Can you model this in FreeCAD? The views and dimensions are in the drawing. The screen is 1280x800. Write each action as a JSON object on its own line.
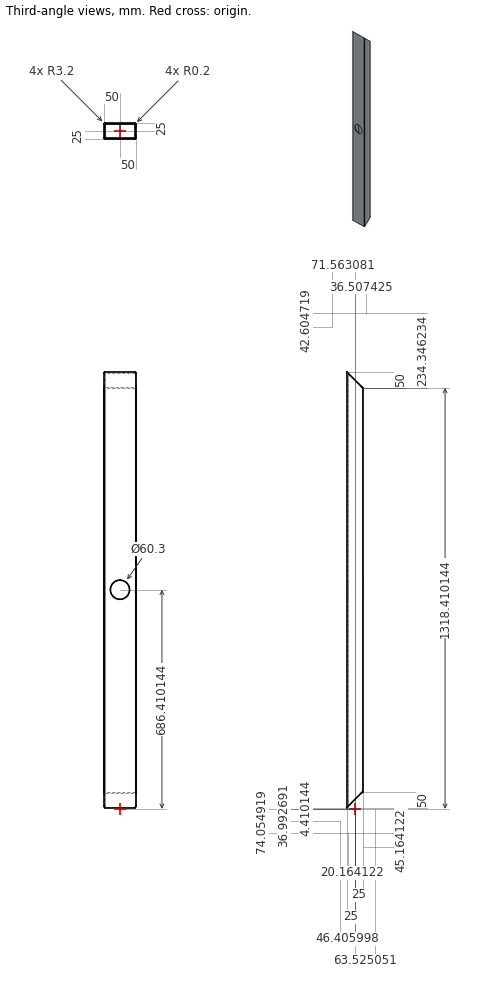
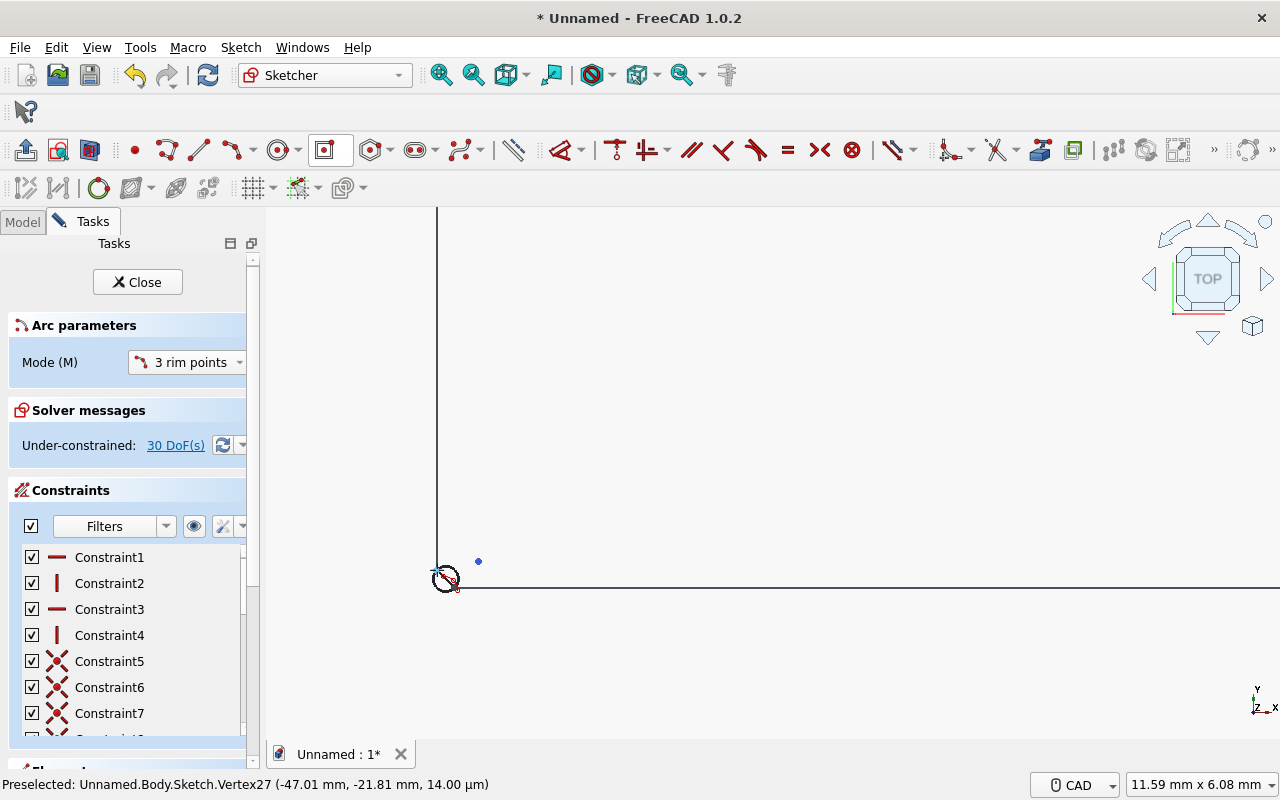
{"action": "scroll", "coordinate": [442, 582], "scroll_direction": "up", "scroll_amount": 6}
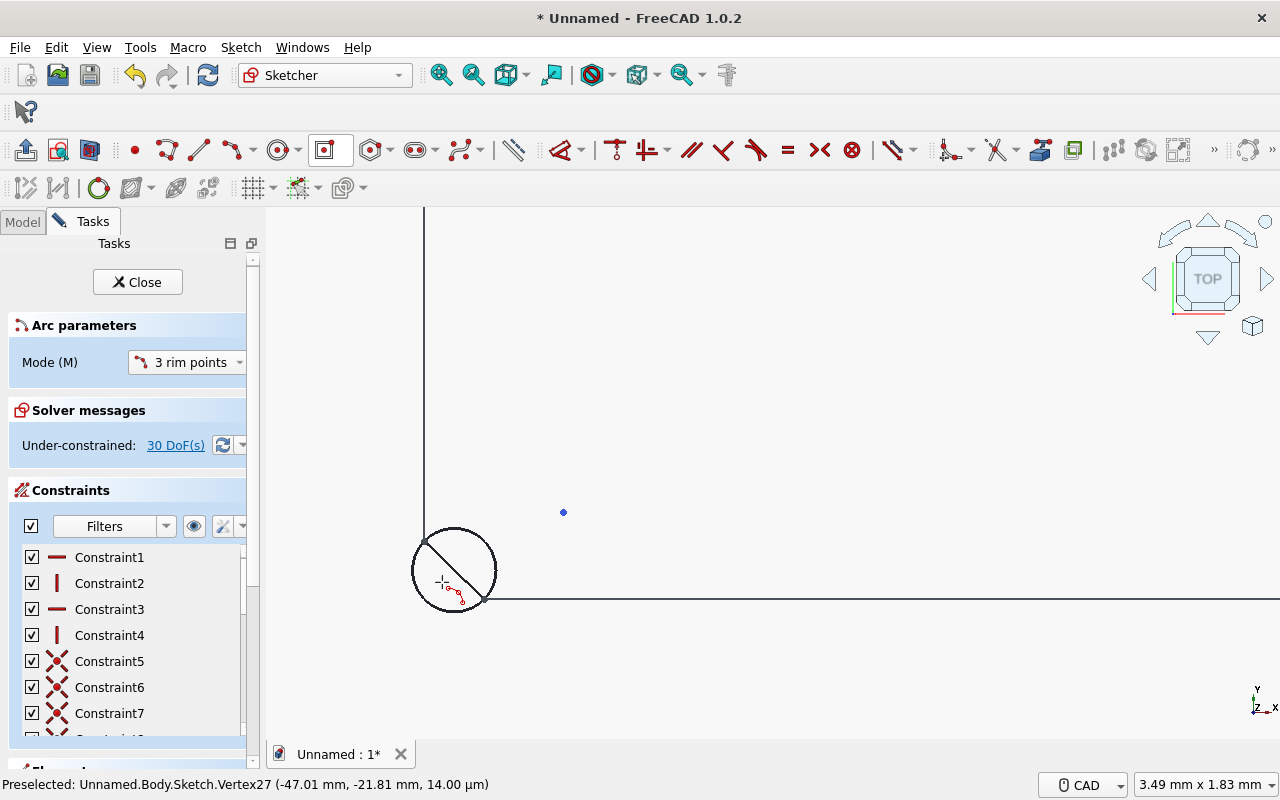
{"action": "left_click", "coordinate": [443, 579]}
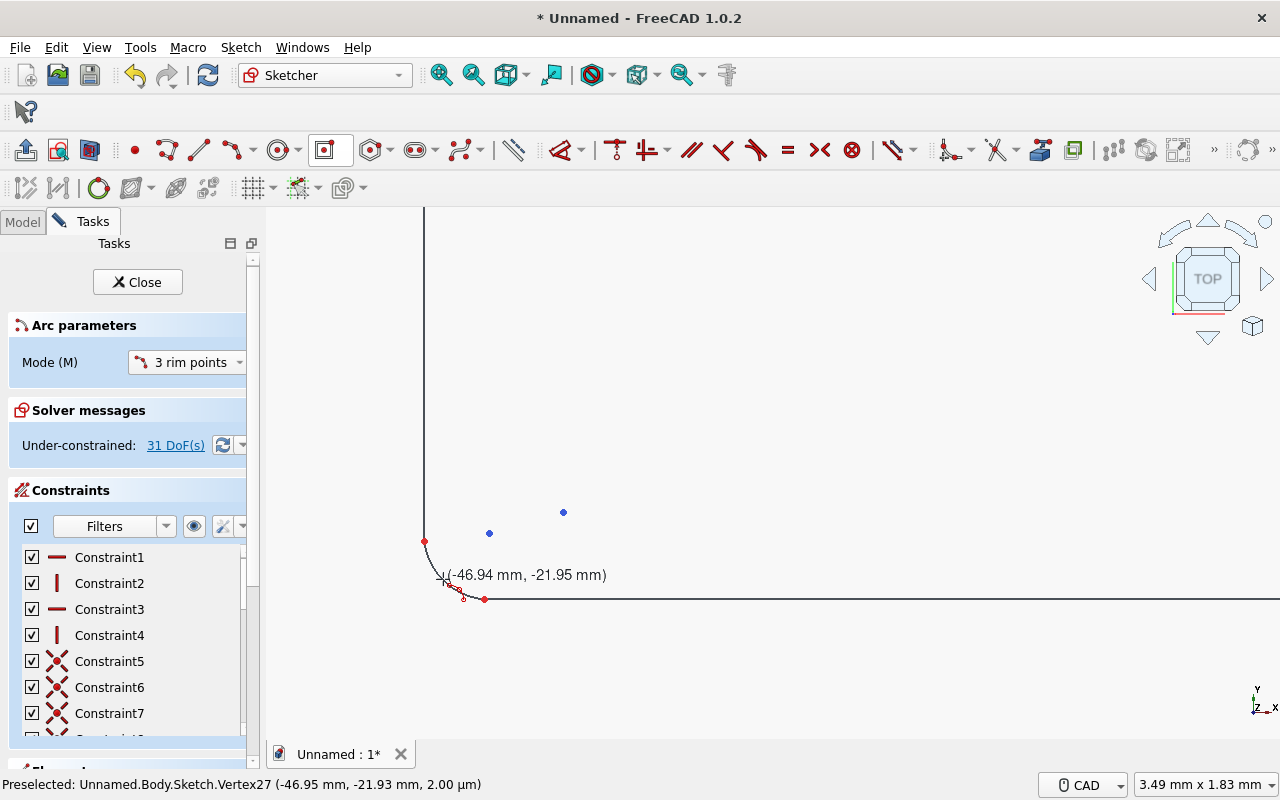
{"action": "scroll", "coordinate": [704, 473], "scroll_direction": "down", "scroll_amount": 15}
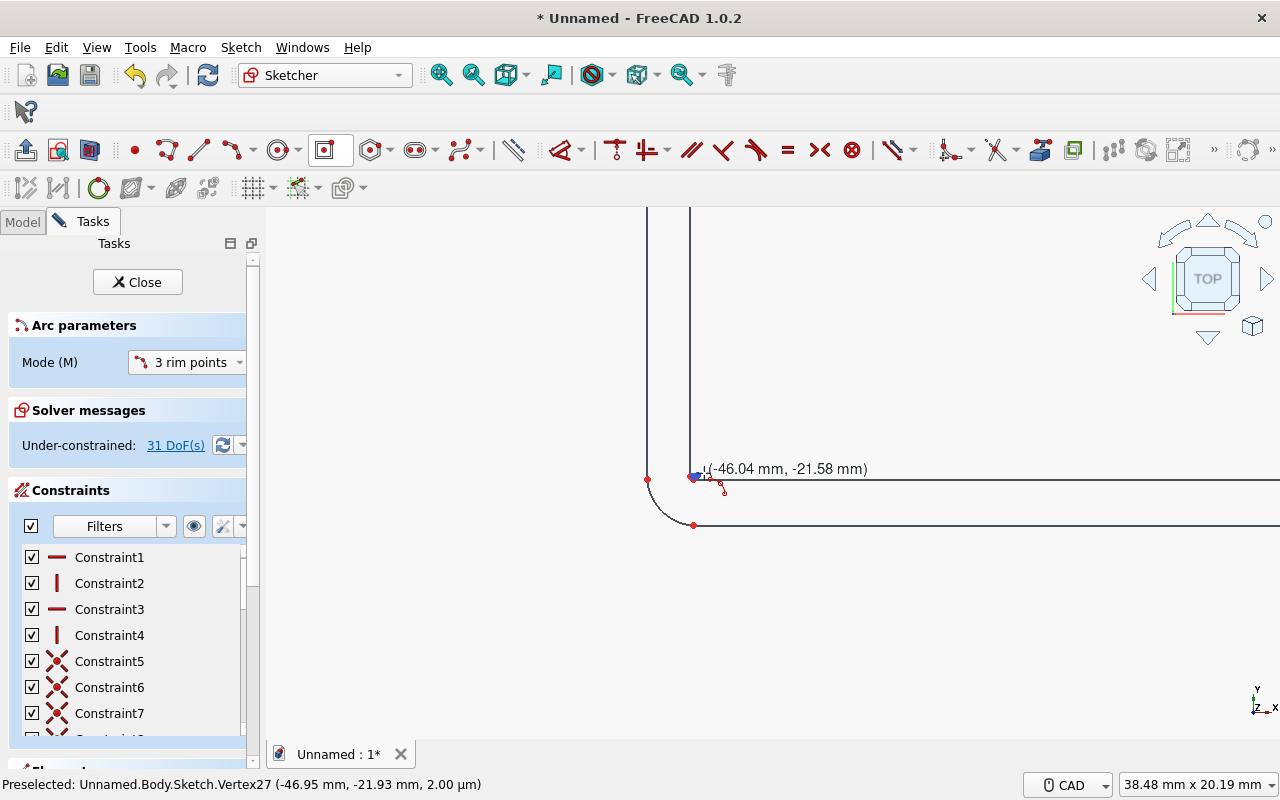
{"action": "scroll", "coordinate": [317, 654], "scroll_direction": "down", "scroll_amount": 5}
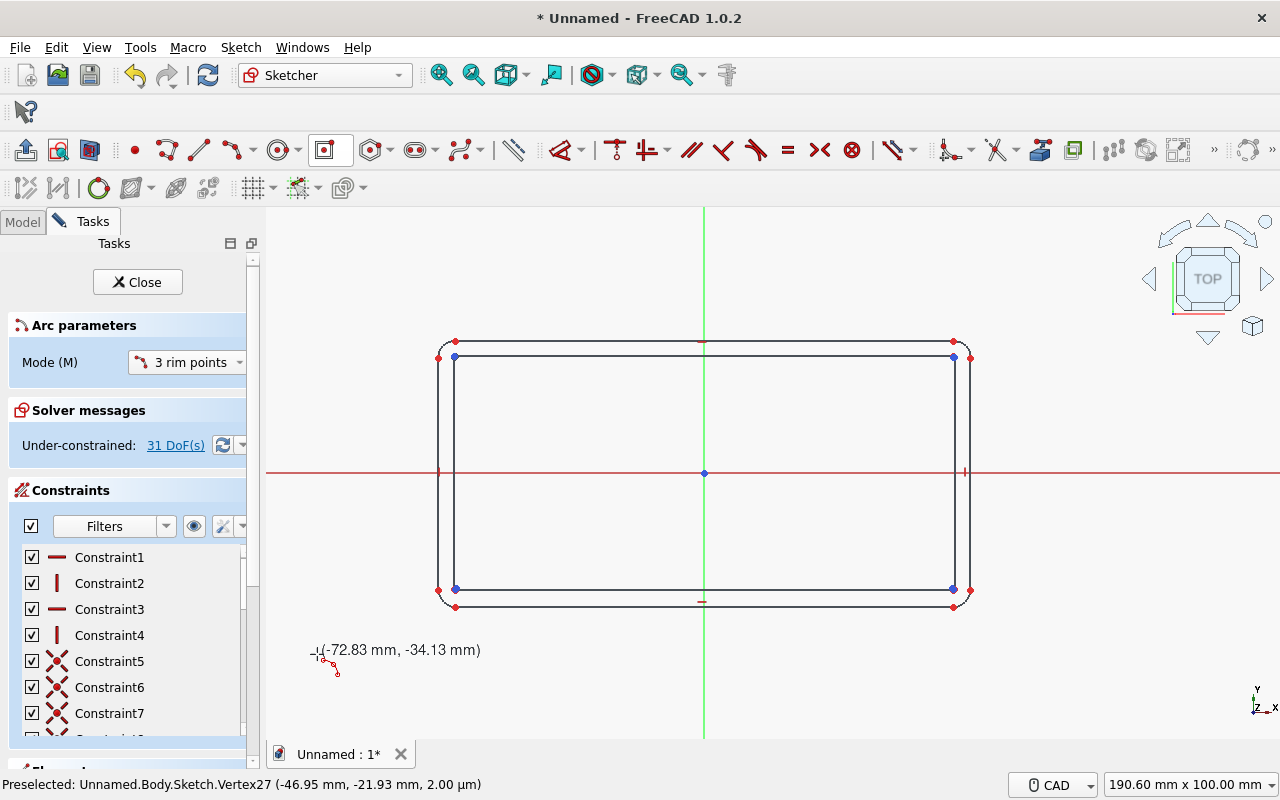
{"action": "scroll", "coordinate": [454, 357], "scroll_direction": "up", "scroll_amount": 14}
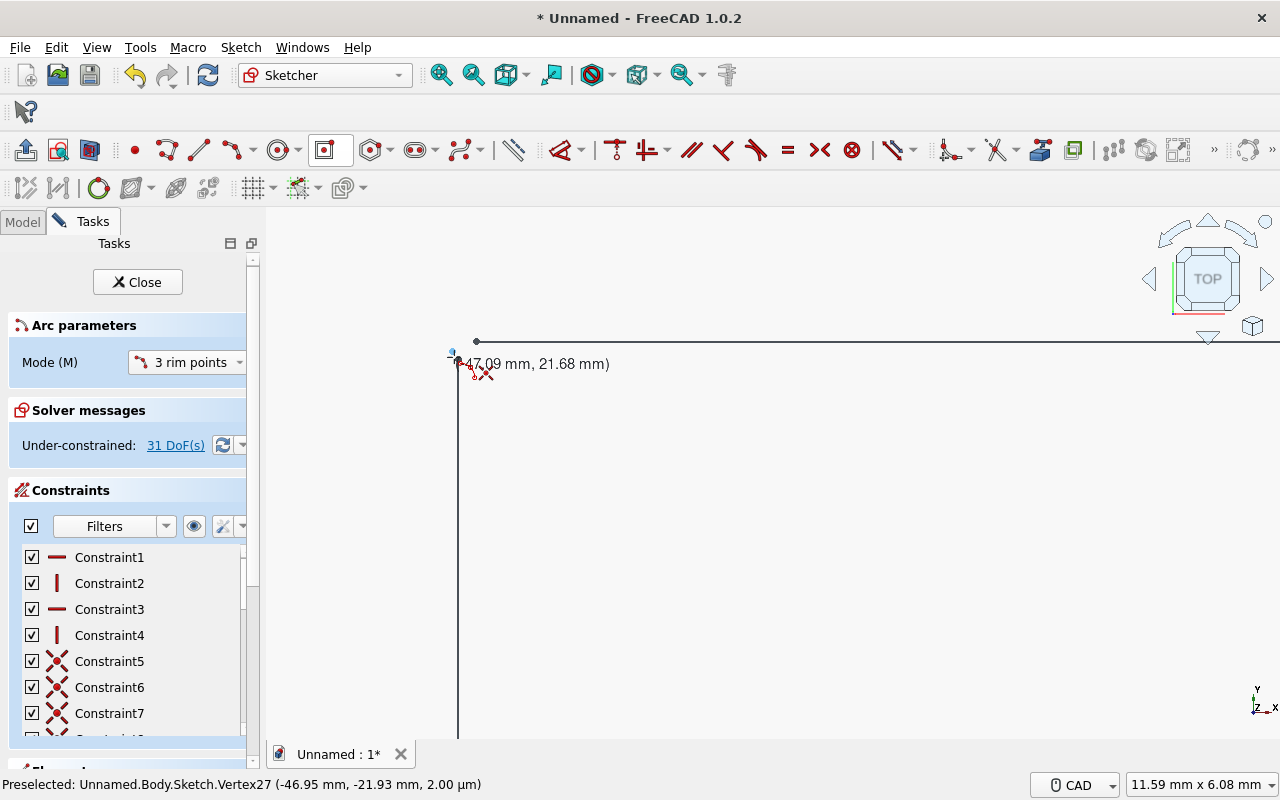
{"action": "left_click", "coordinate": [458, 359]}
{"action": "left_click", "coordinate": [476, 342]}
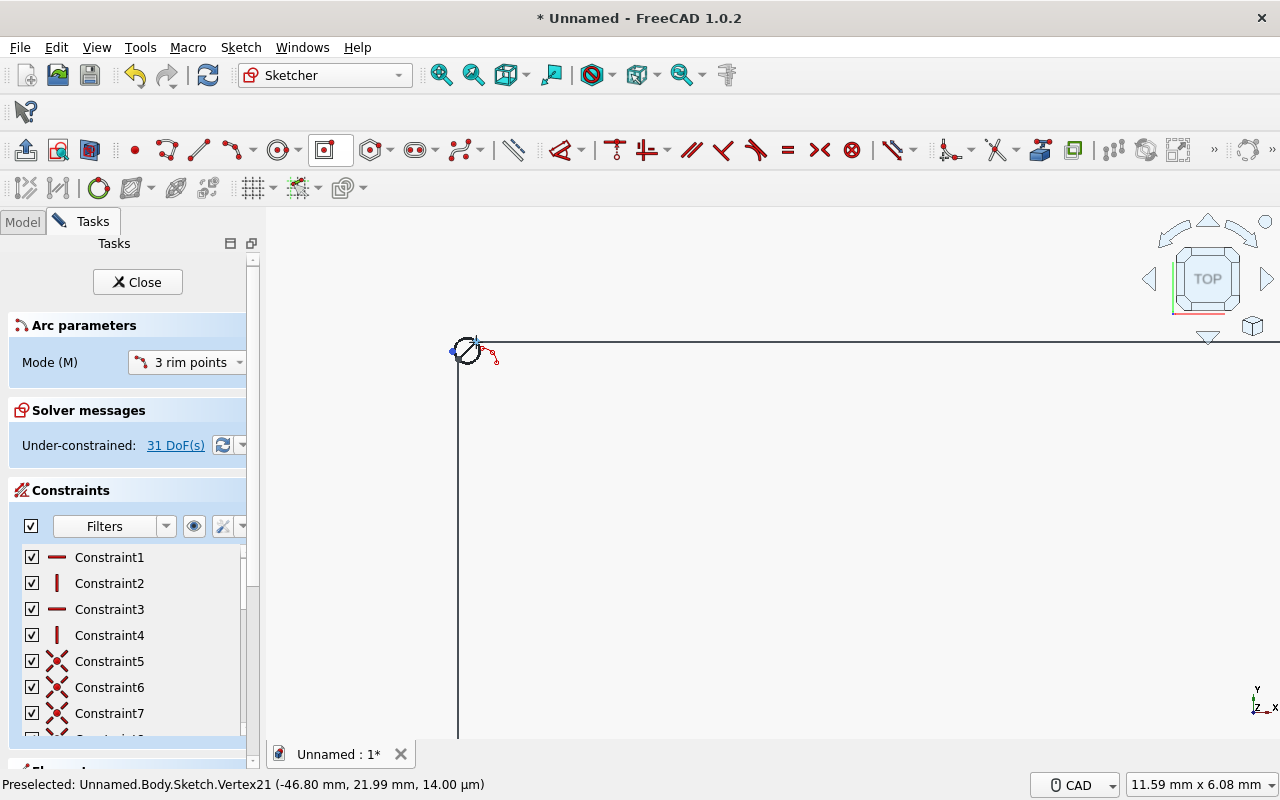
{"action": "scroll", "coordinate": [464, 346], "scroll_direction": "up", "scroll_amount": 6}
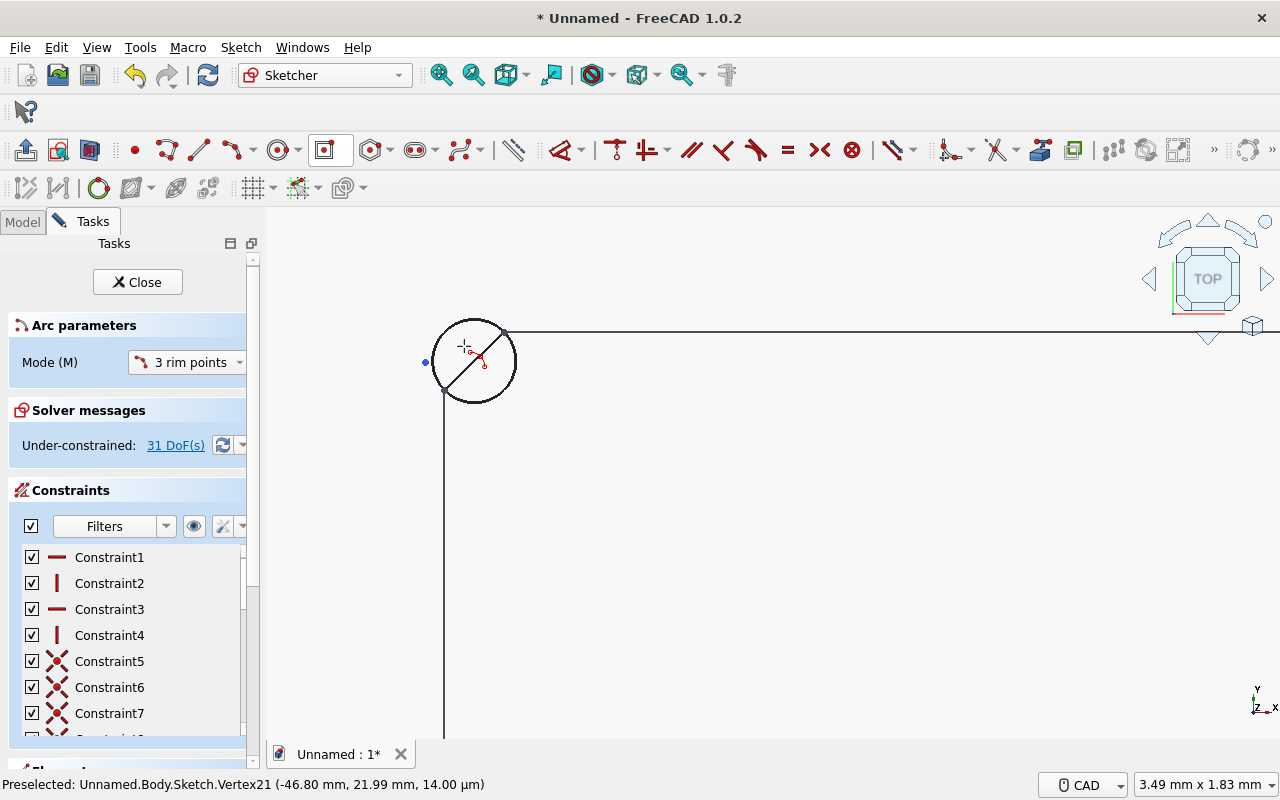
{"action": "left_click", "coordinate": [463, 346]}
{"action": "key", "text": "Escape"}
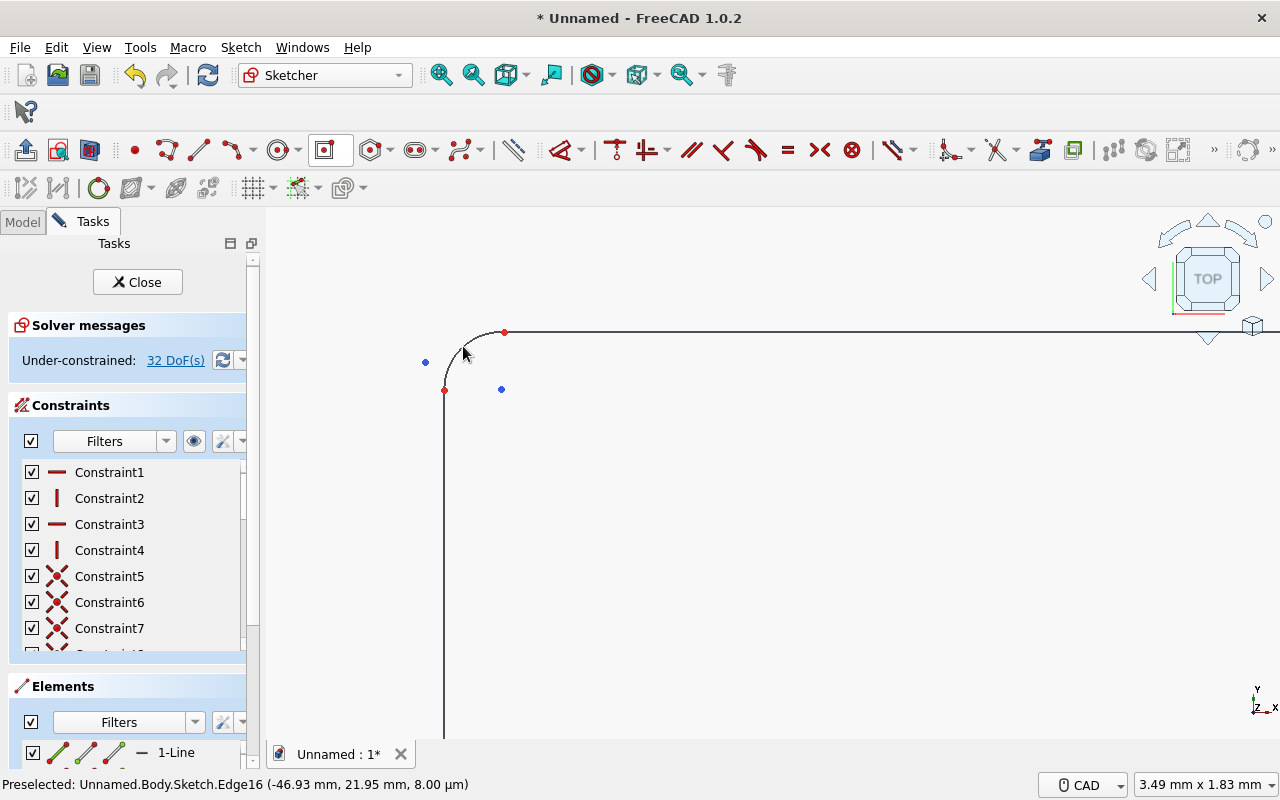
{"action": "scroll", "coordinate": [704, 473], "scroll_direction": "down", "scroll_amount": 15}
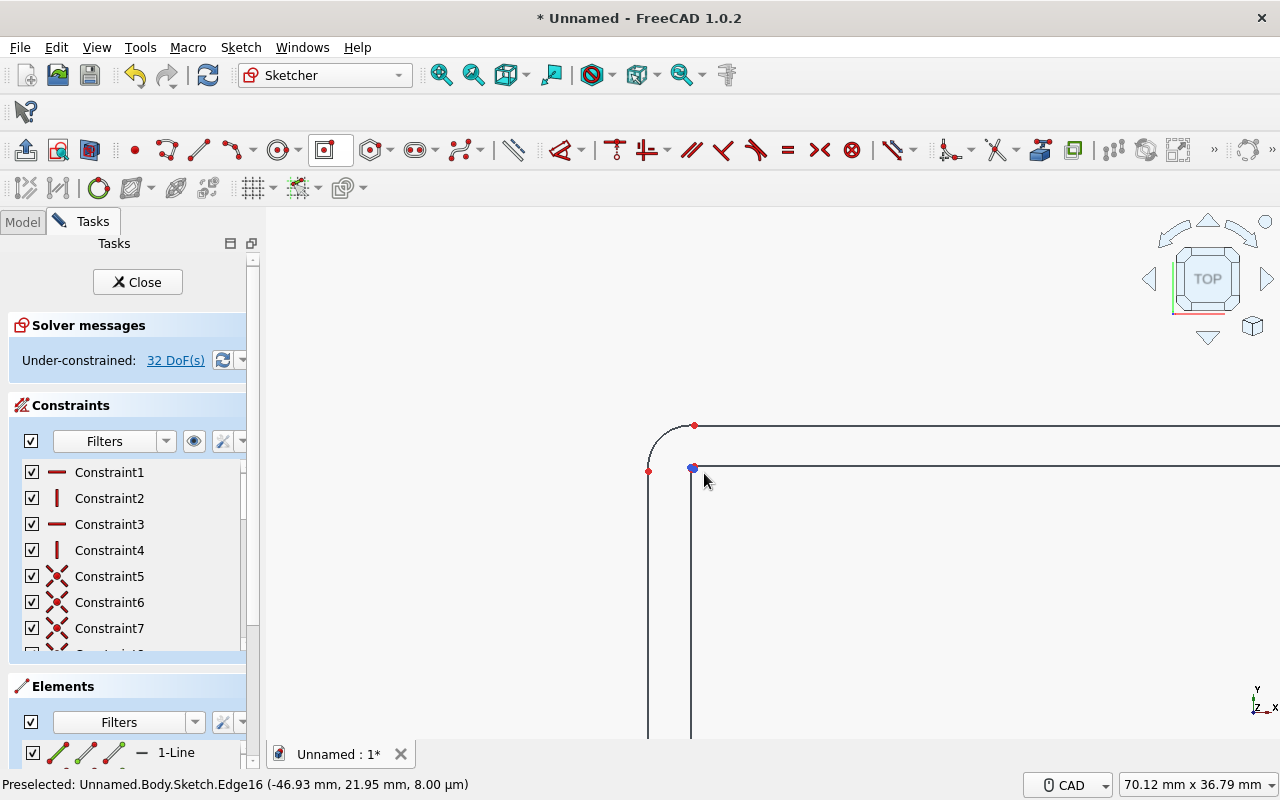
{"action": "scroll", "coordinate": [316, 292], "scroll_direction": "down", "scroll_amount": 5}